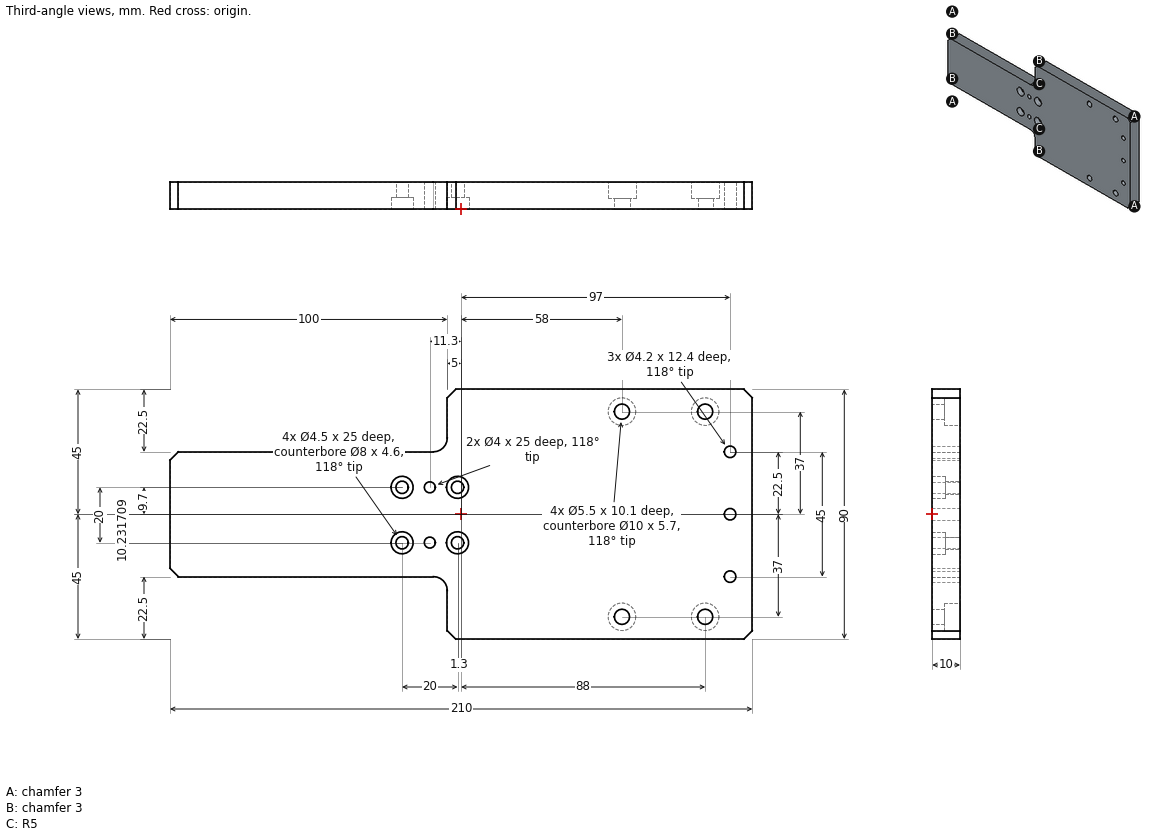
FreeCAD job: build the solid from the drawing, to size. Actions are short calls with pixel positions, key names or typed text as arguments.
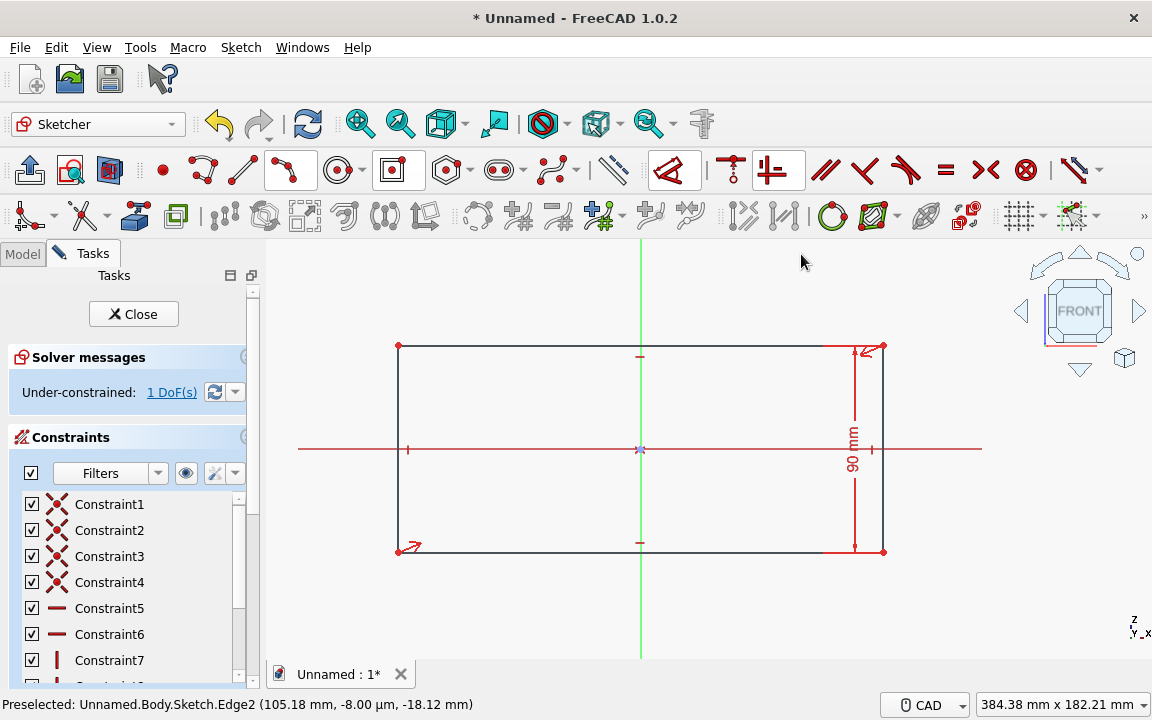
click(544, 553)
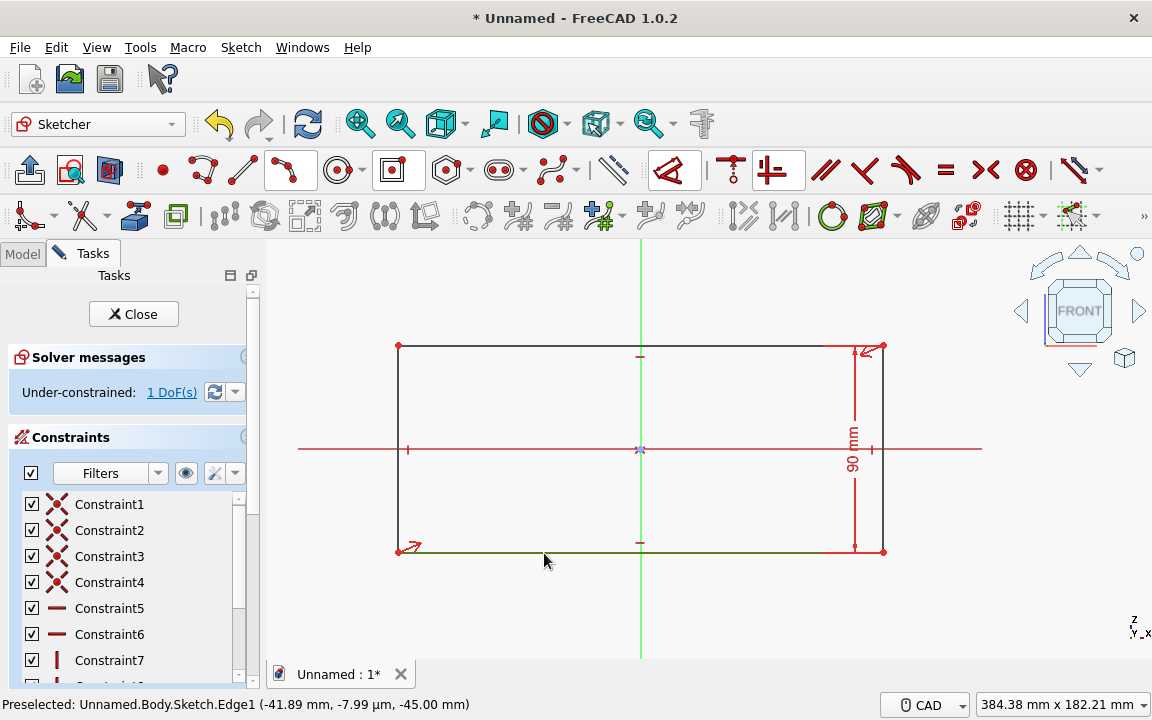
click(696, 170)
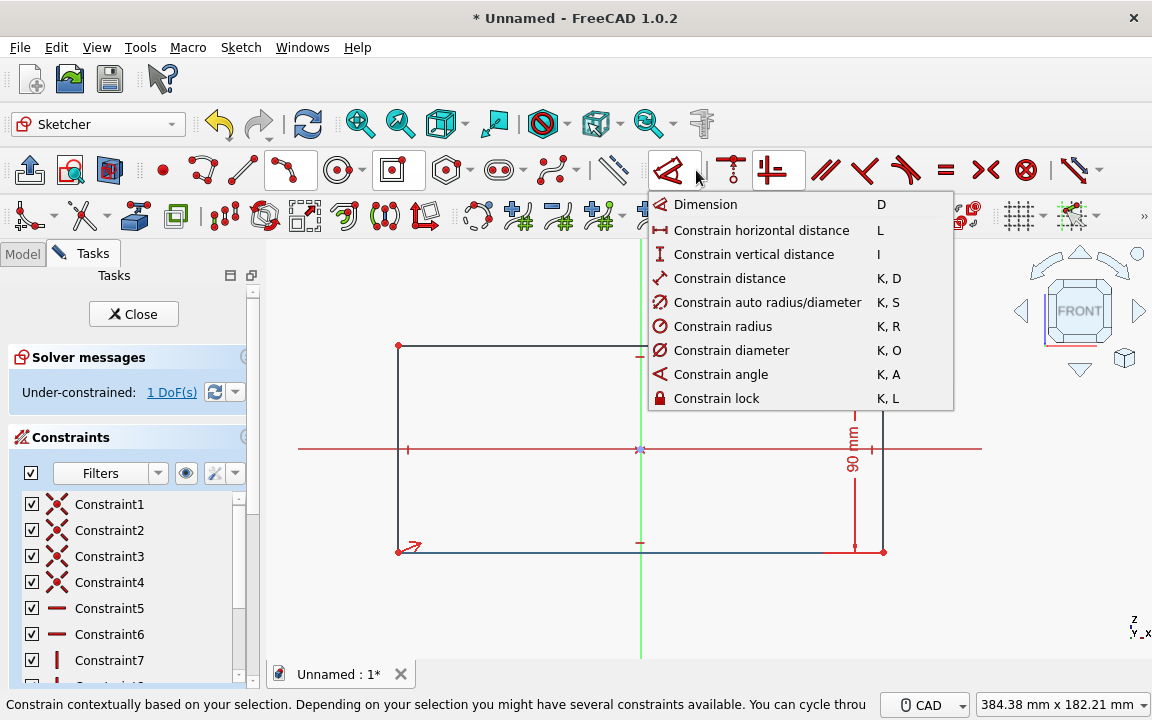
click(801, 230)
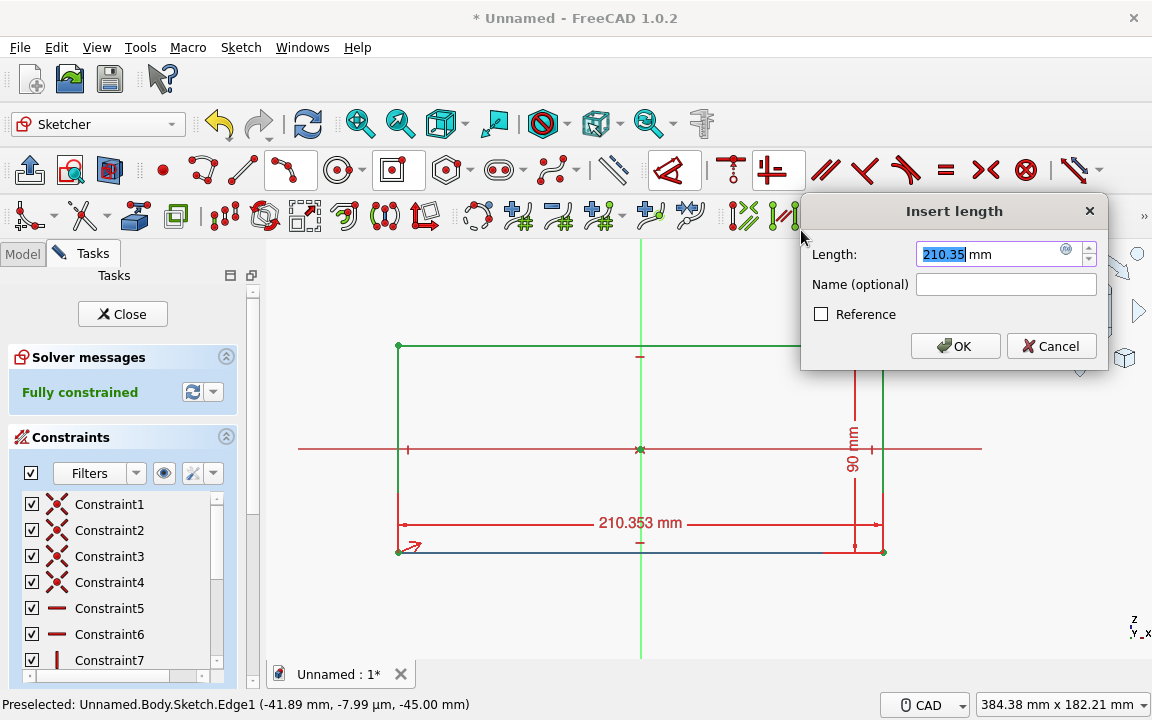
text(210)
key(Return)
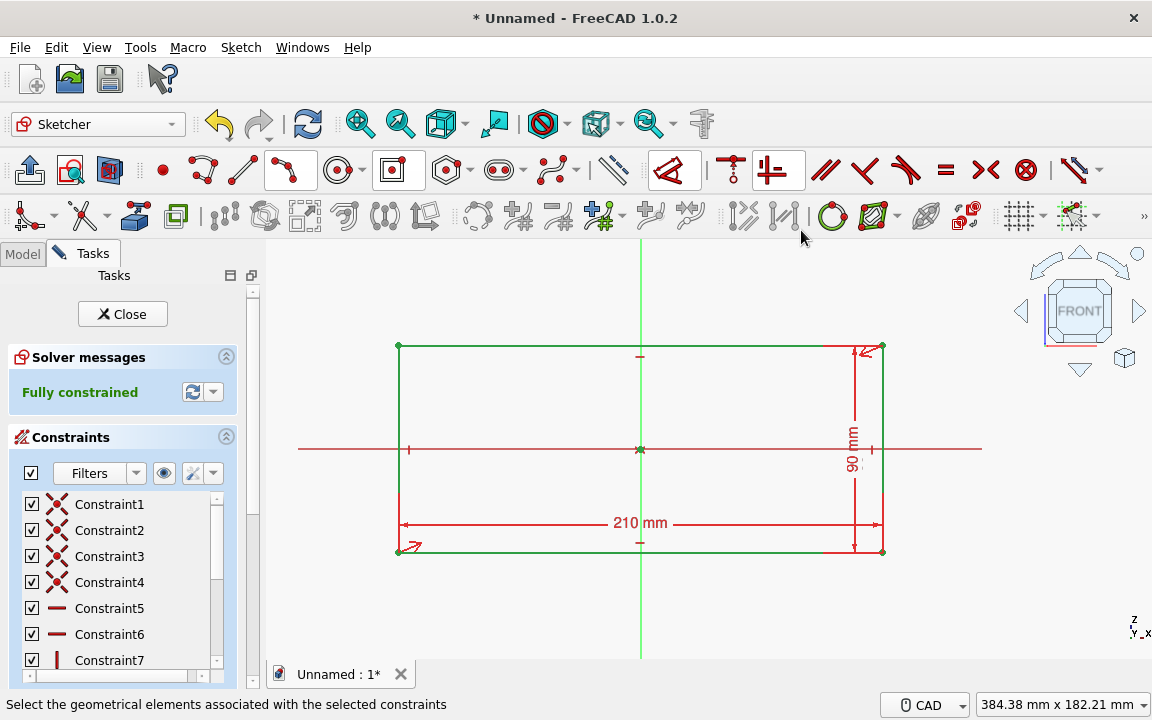
click(123, 314)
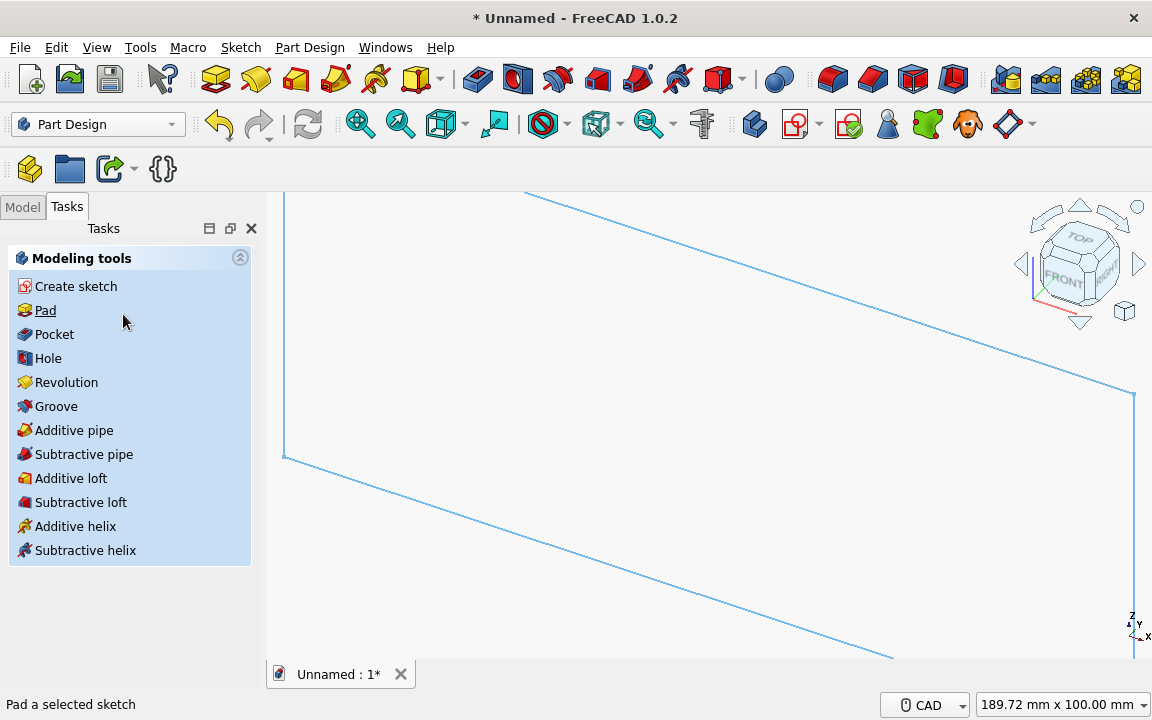
click(216, 80)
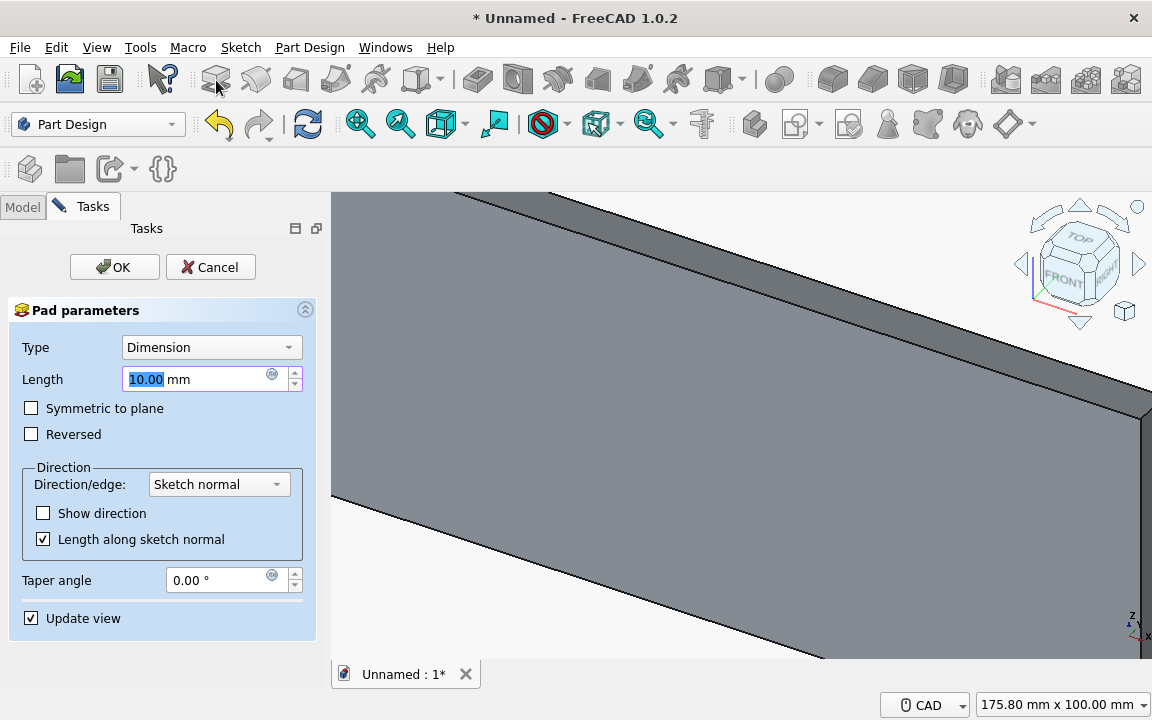
text(10)
key(Tab)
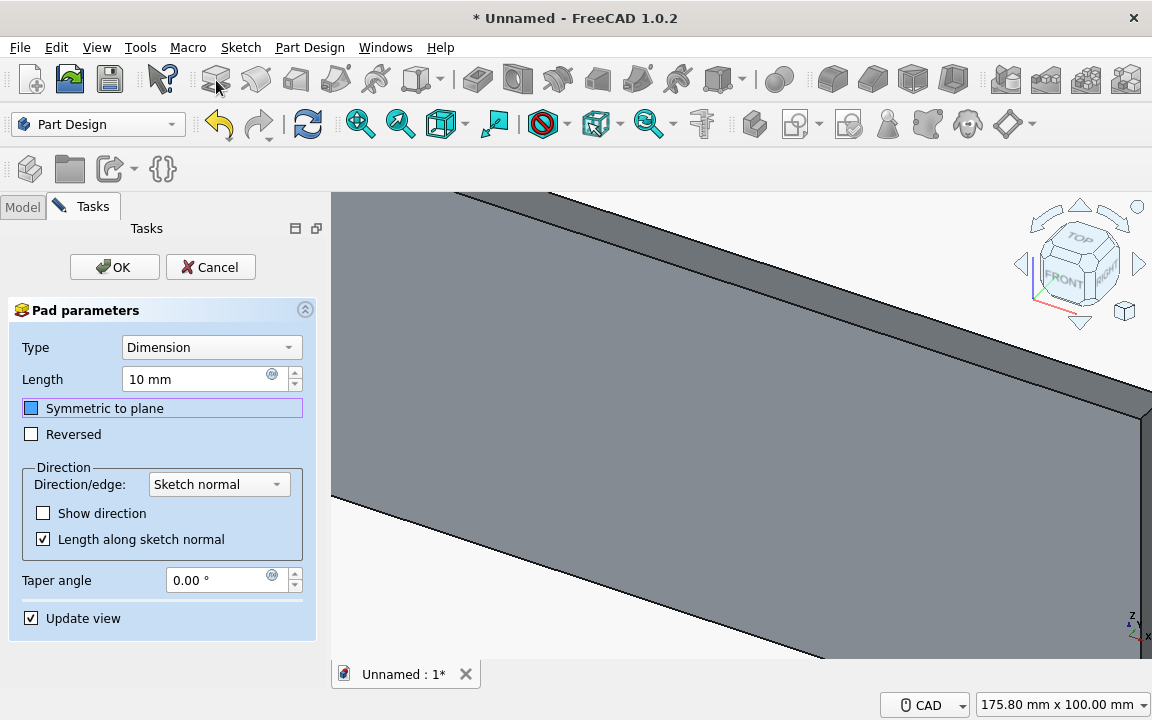
click(30, 434)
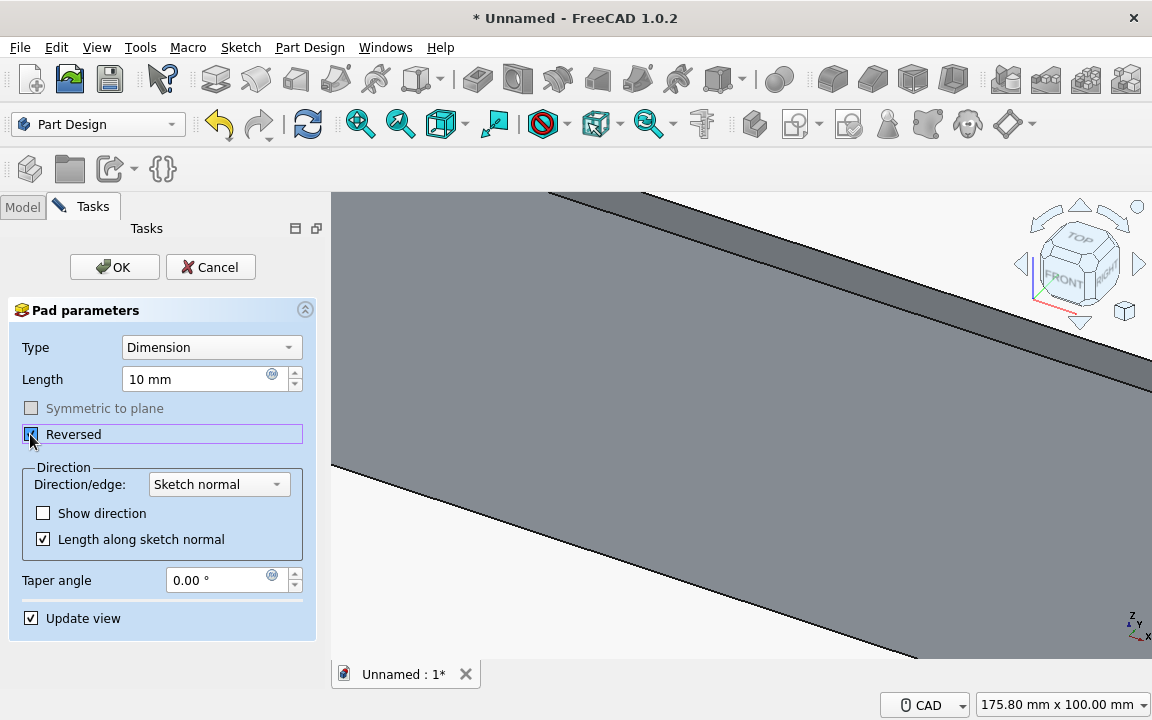
click(115, 267)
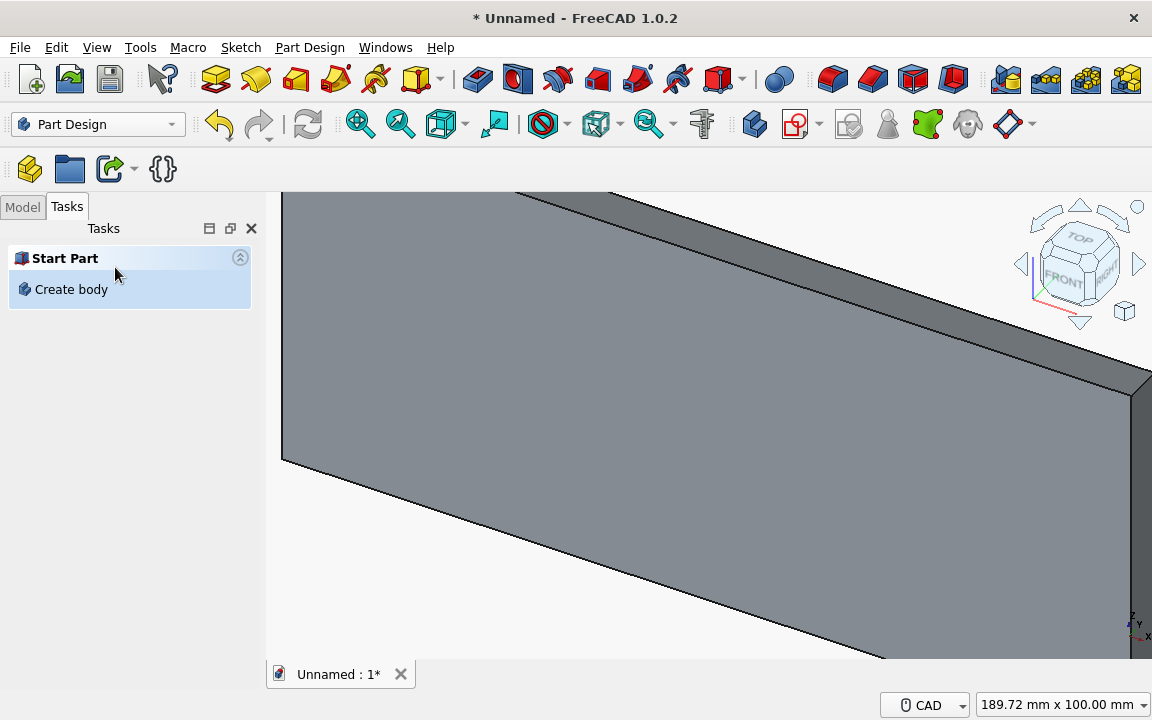
click(362, 124)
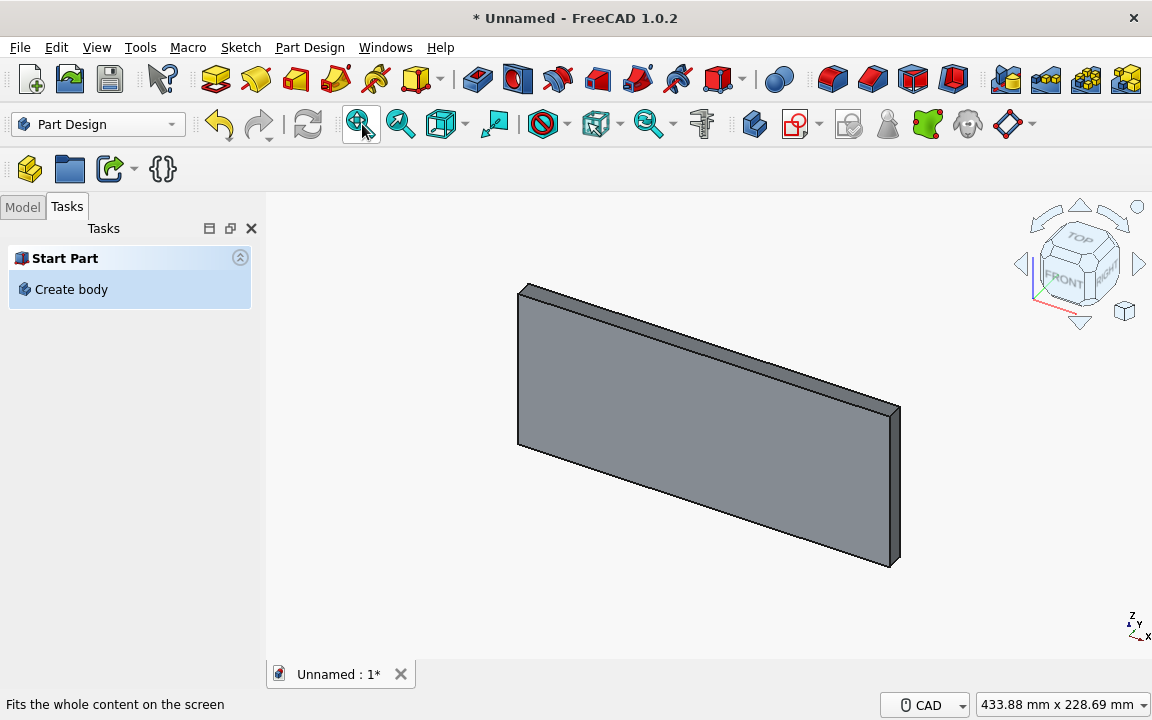
click(895, 411)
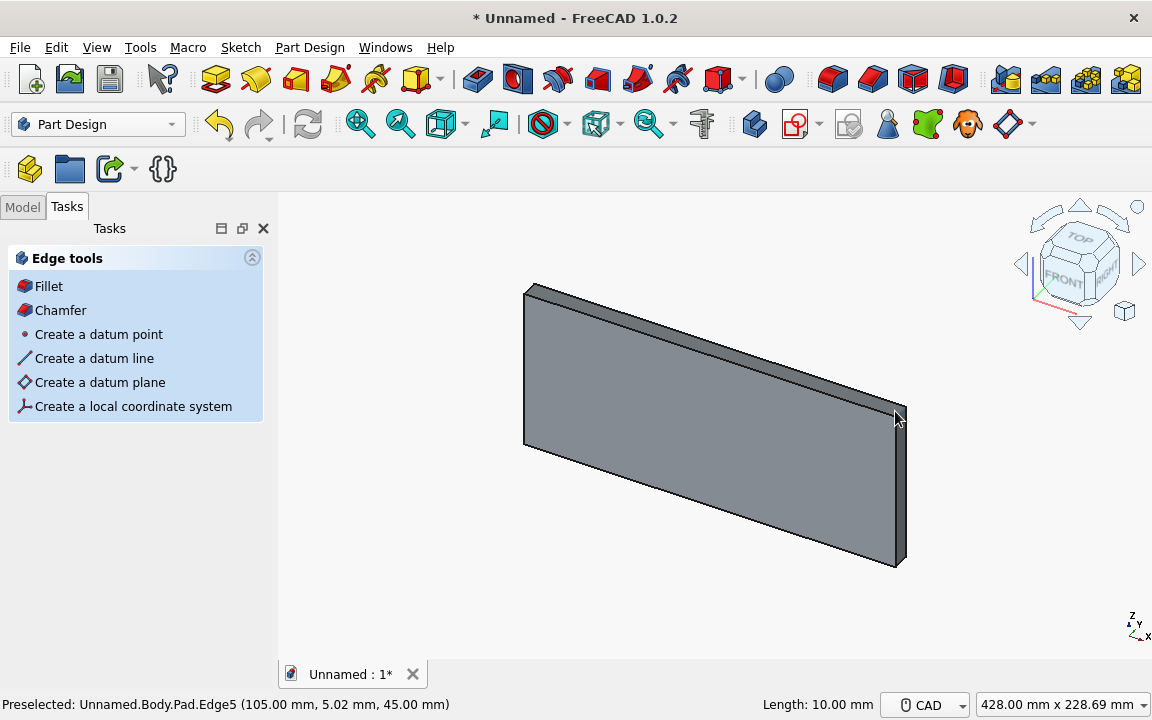
scroll(529, 288, up, 4)